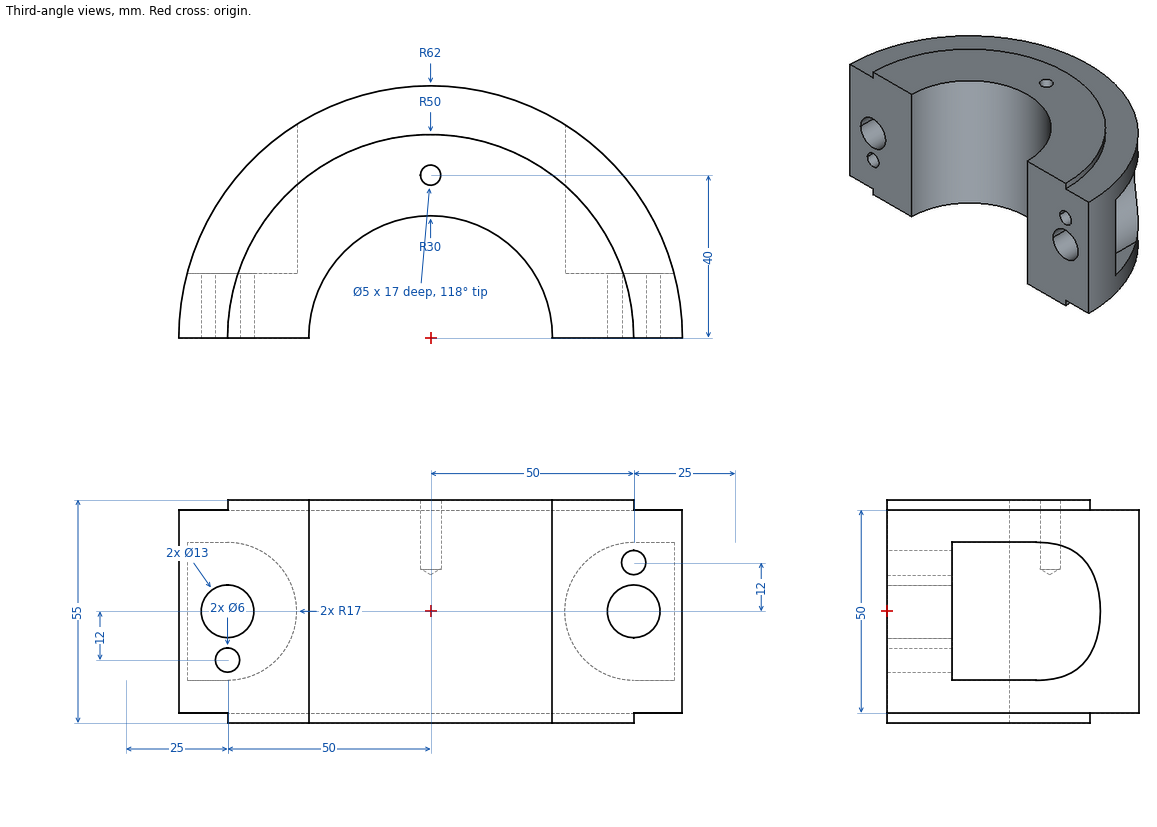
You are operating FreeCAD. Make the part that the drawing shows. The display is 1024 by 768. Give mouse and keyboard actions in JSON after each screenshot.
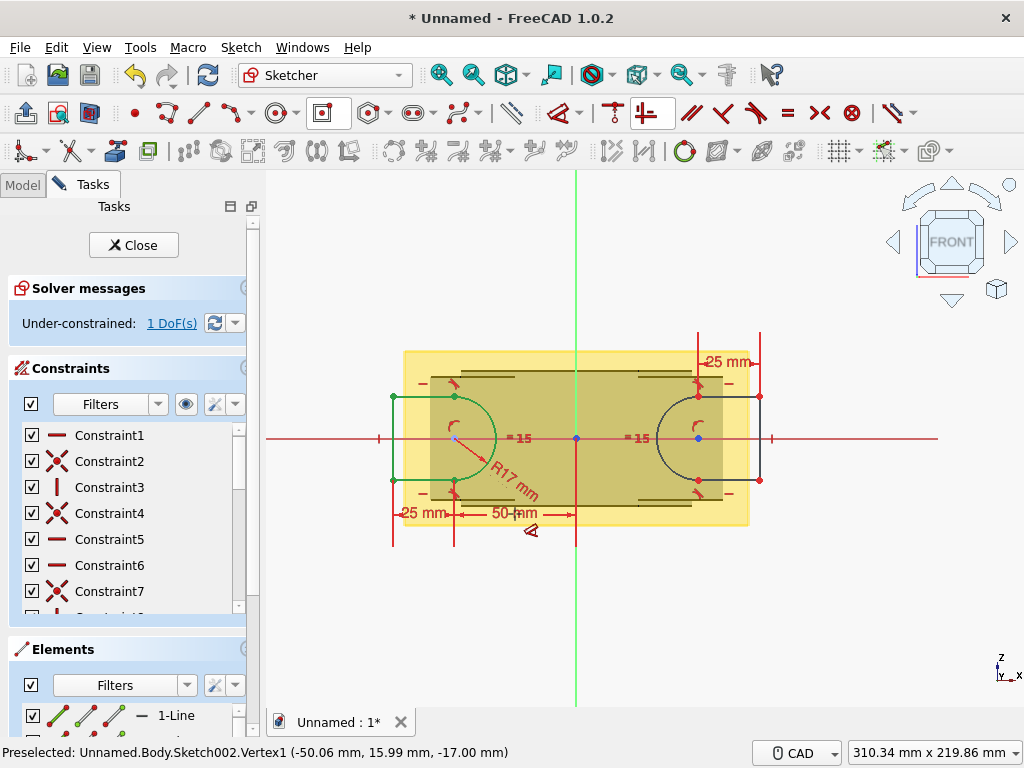
{"action": "left_click", "coordinate": [699, 397]}
{"action": "left_click", "coordinate": [638, 363]}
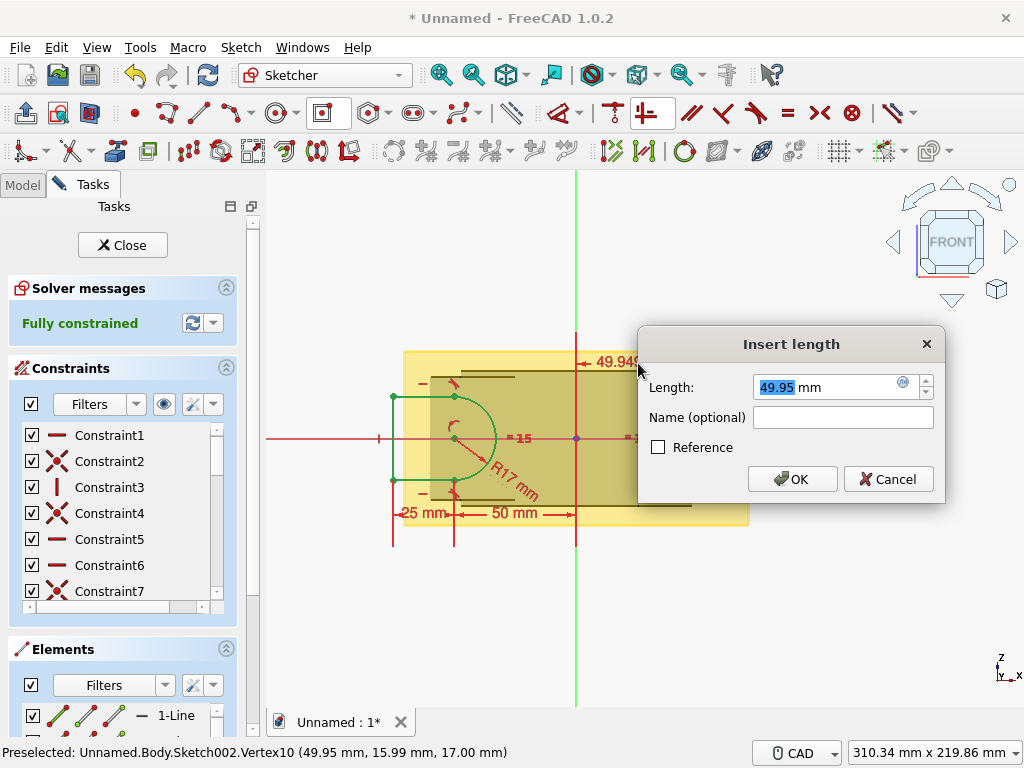
{"action": "type", "text": "50"}
{"action": "key", "text": "Return"}
{"action": "key", "text": "Escape"}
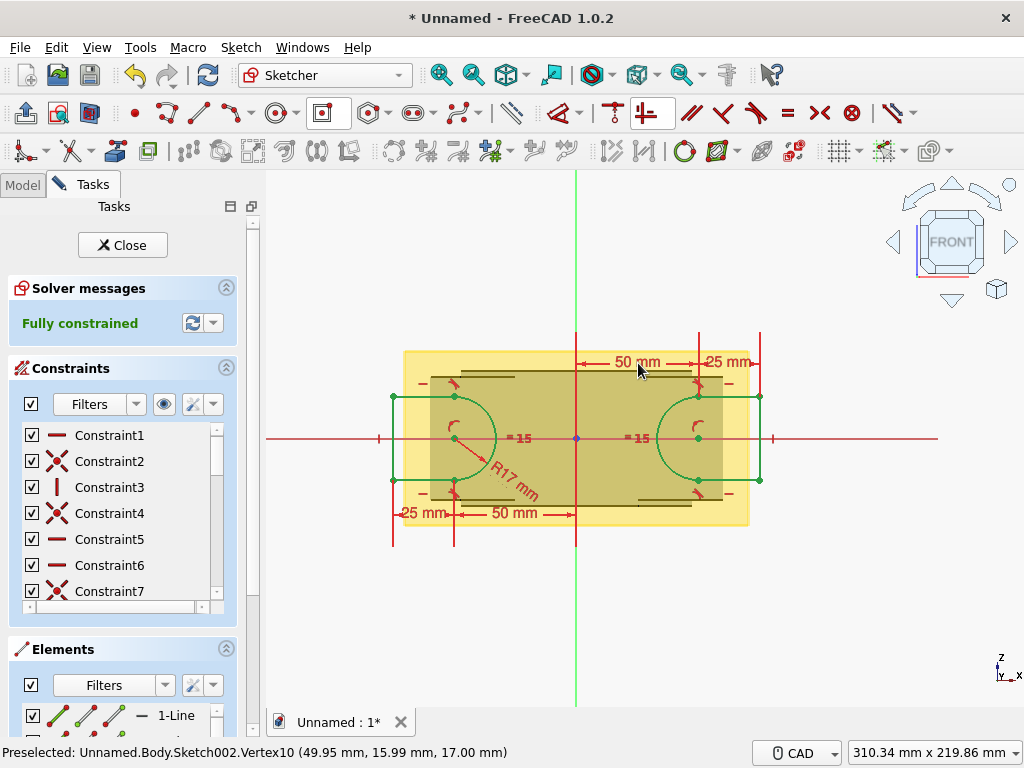
{"action": "left_click", "coordinate": [123, 245]}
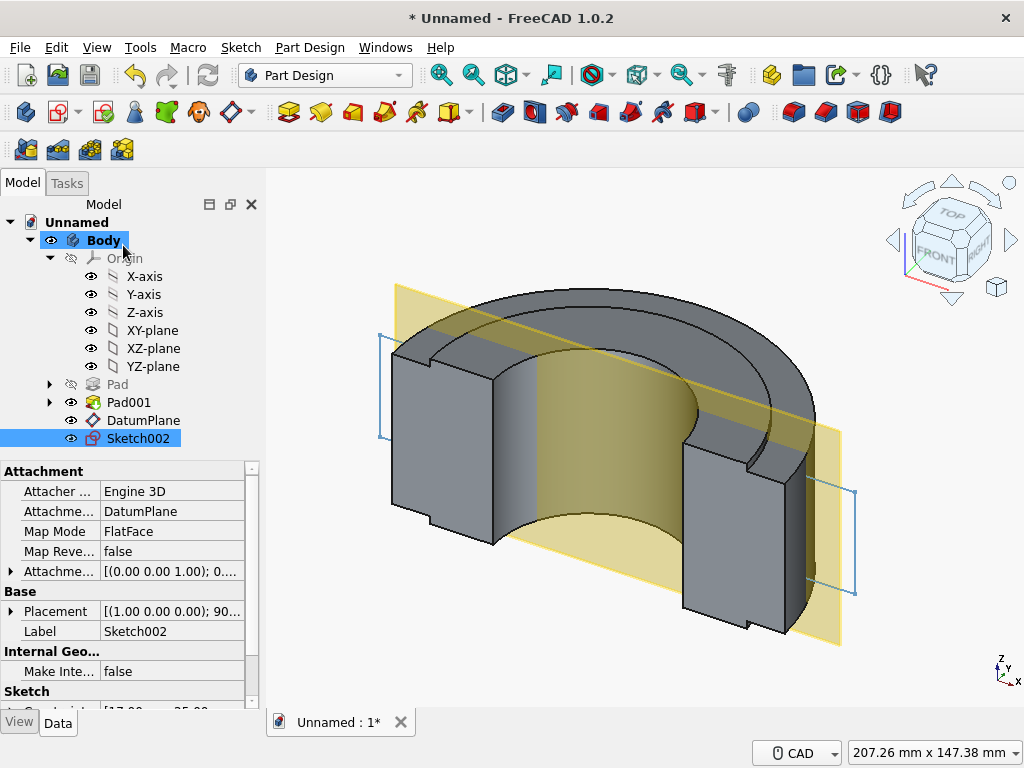
{"action": "left_click", "coordinate": [504, 112]}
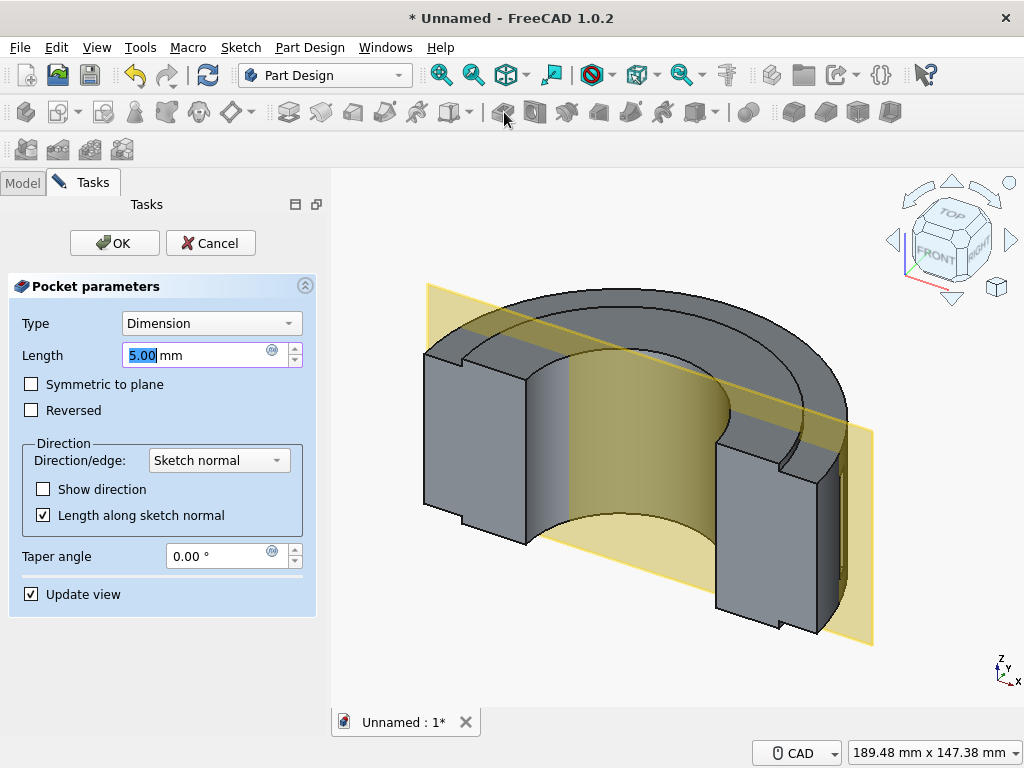
{"action": "left_click", "coordinate": [212, 324]}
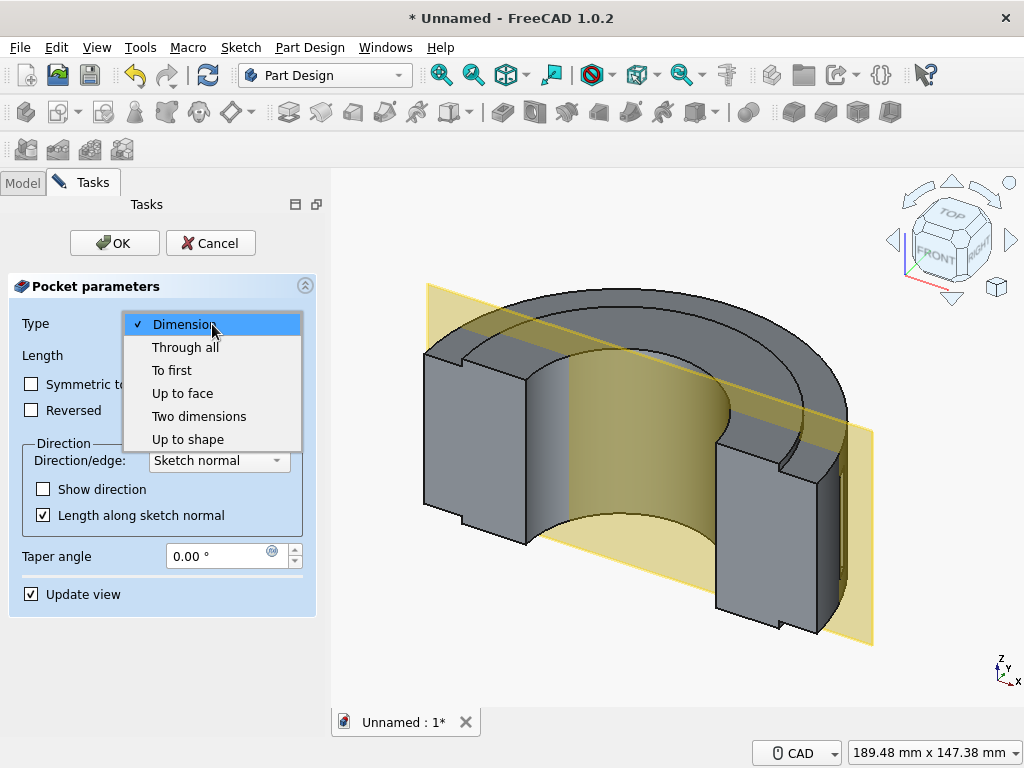
{"action": "left_click", "coordinate": [212, 348]}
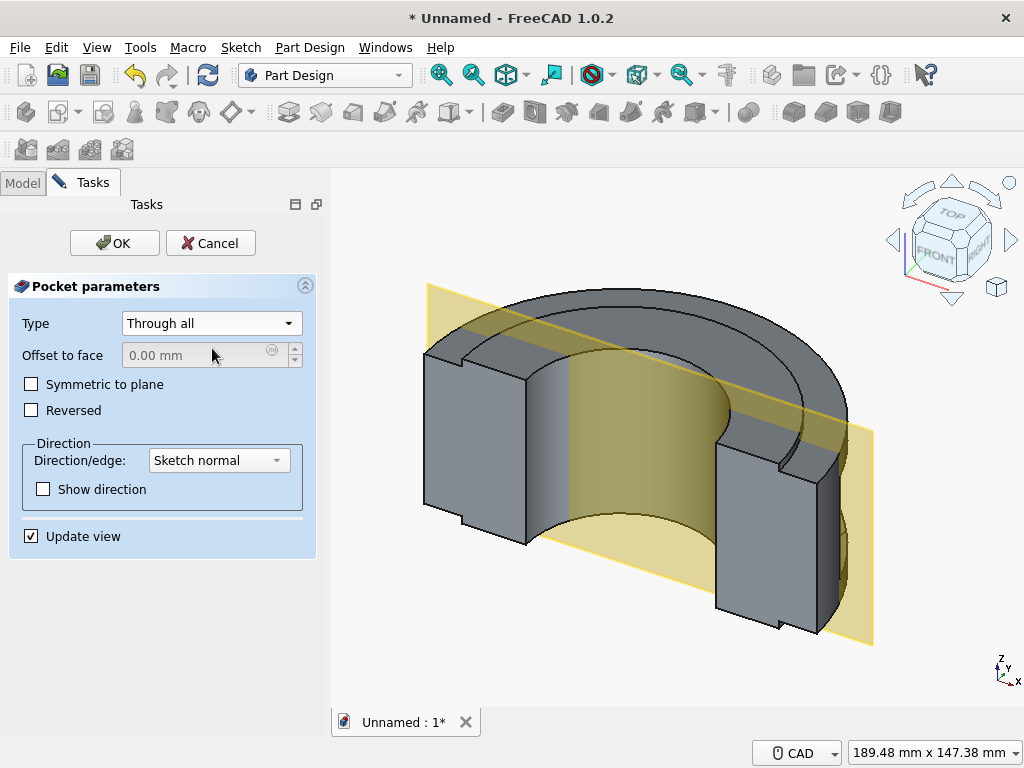
{"action": "left_click", "coordinate": [115, 243]}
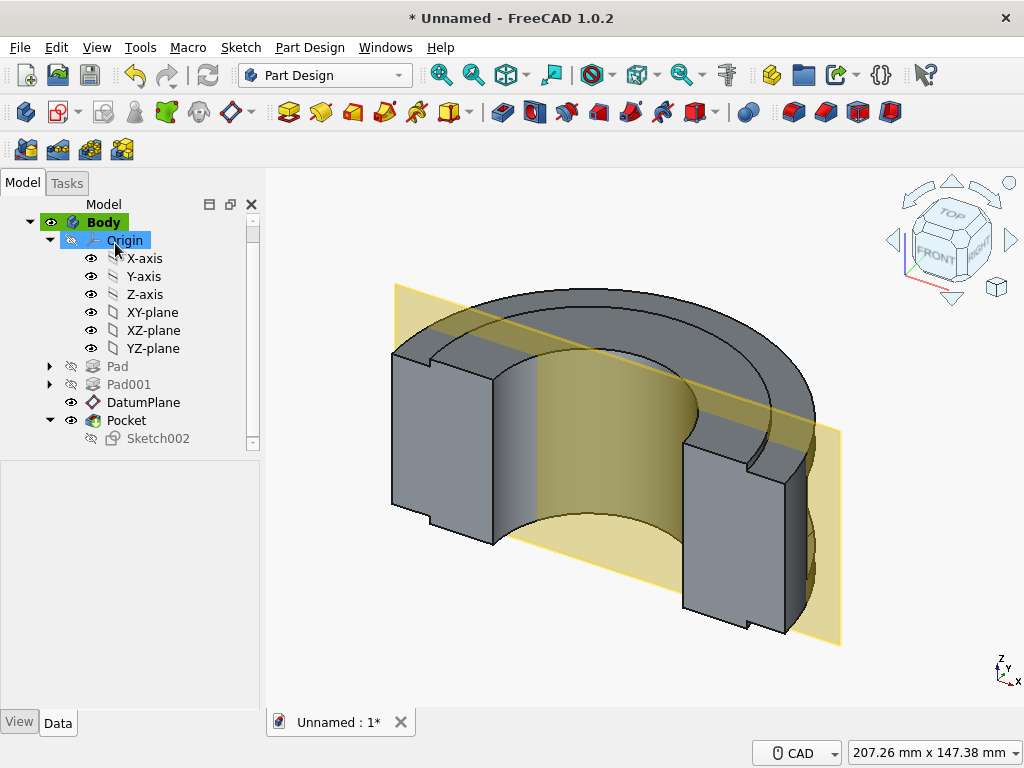
{"action": "left_click", "coordinate": [116, 402]}
{"action": "key", "text": "space"}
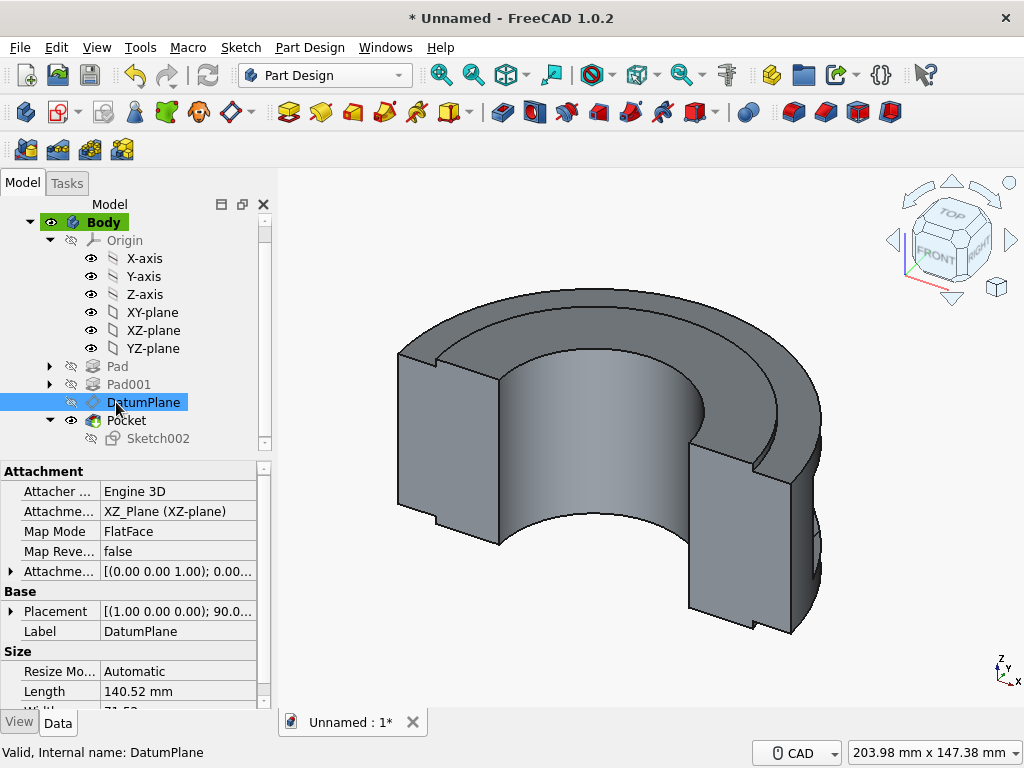
{"action": "key", "text": "4"}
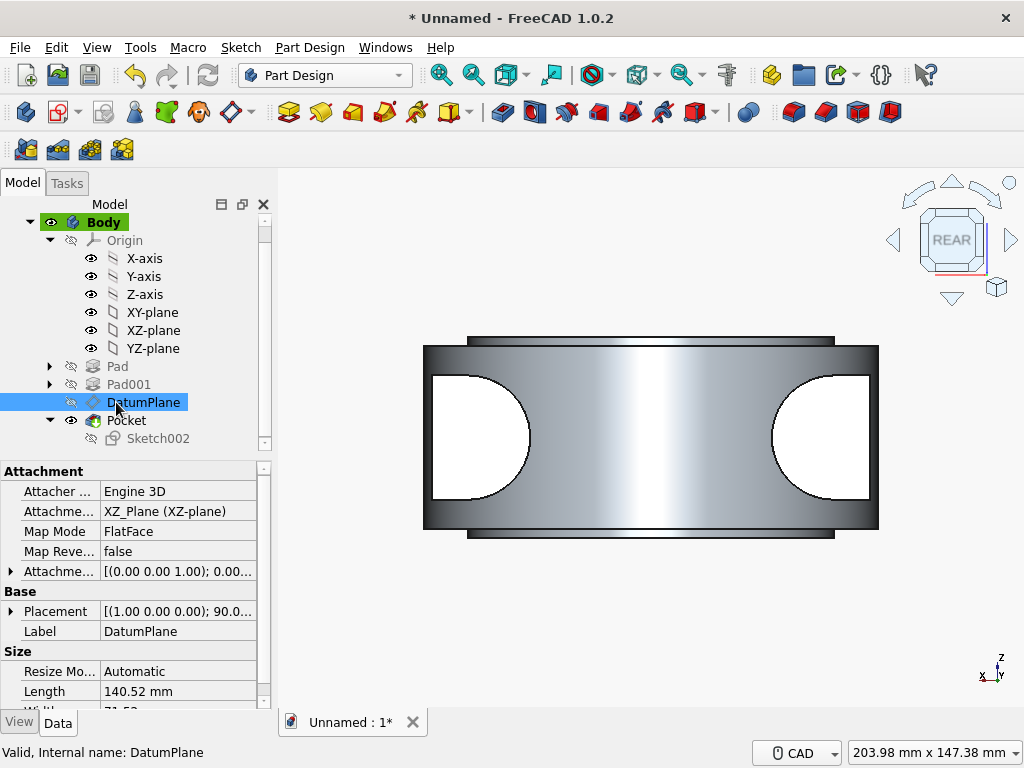
{"action": "left_click", "coordinate": [821, 437]}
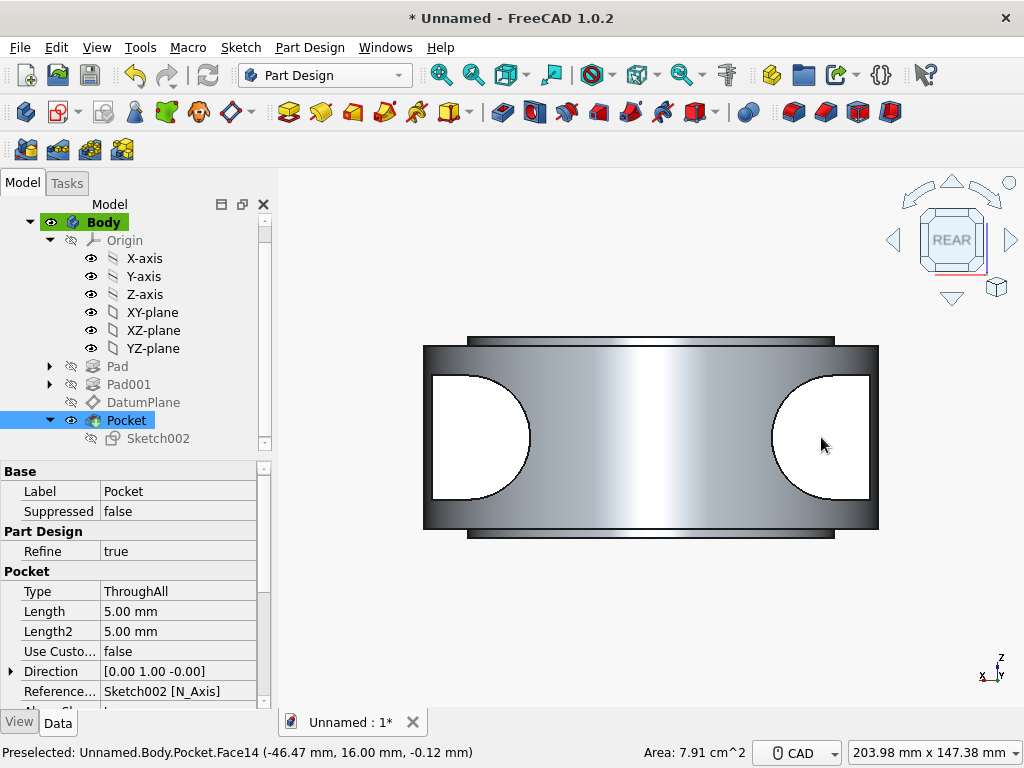
{"action": "left_click", "coordinate": [58, 112]}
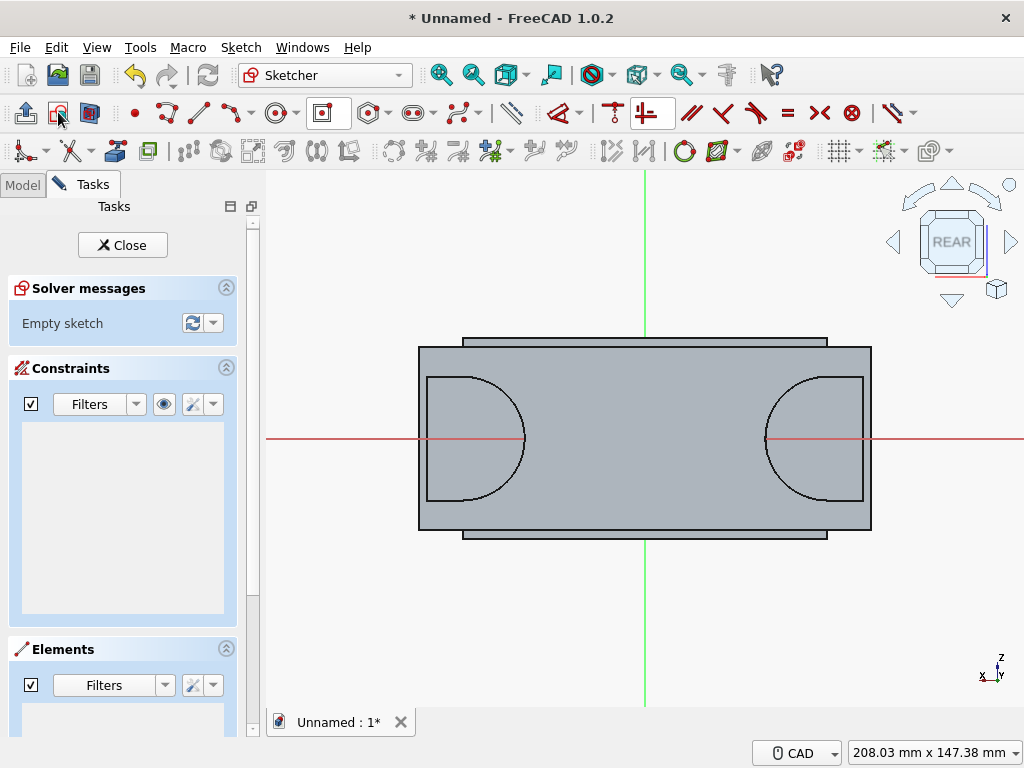
{"action": "scroll", "coordinate": [294, 438], "scroll_direction": "down", "scroll_amount": 1}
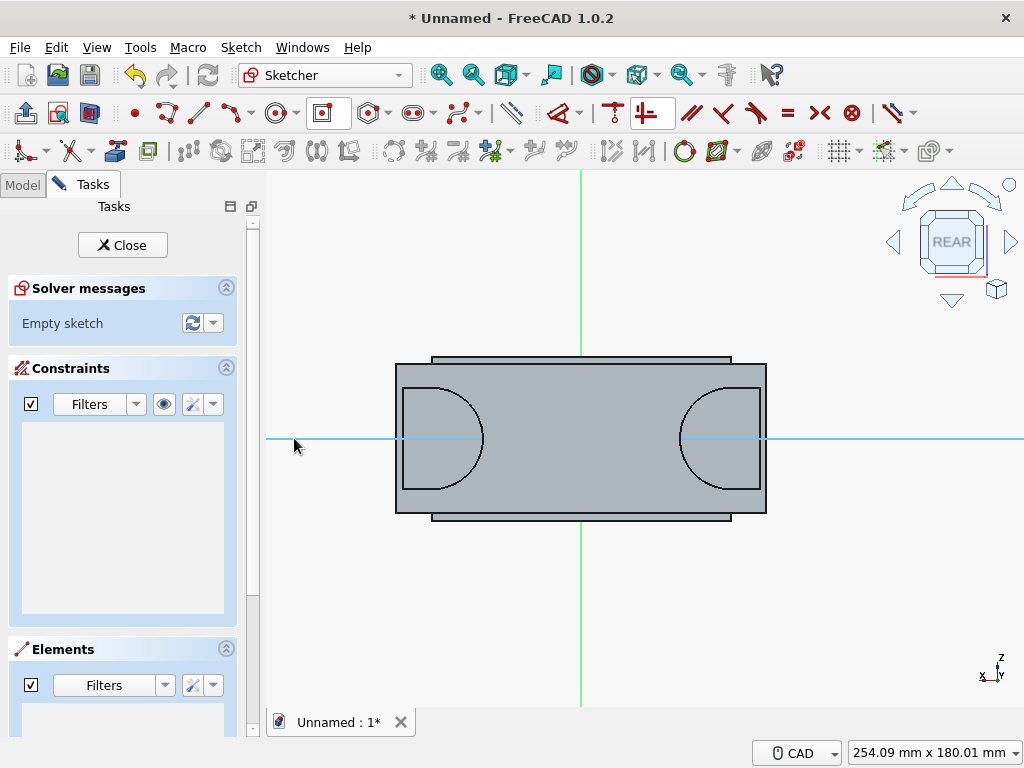
{"action": "left_click", "coordinate": [276, 114]}